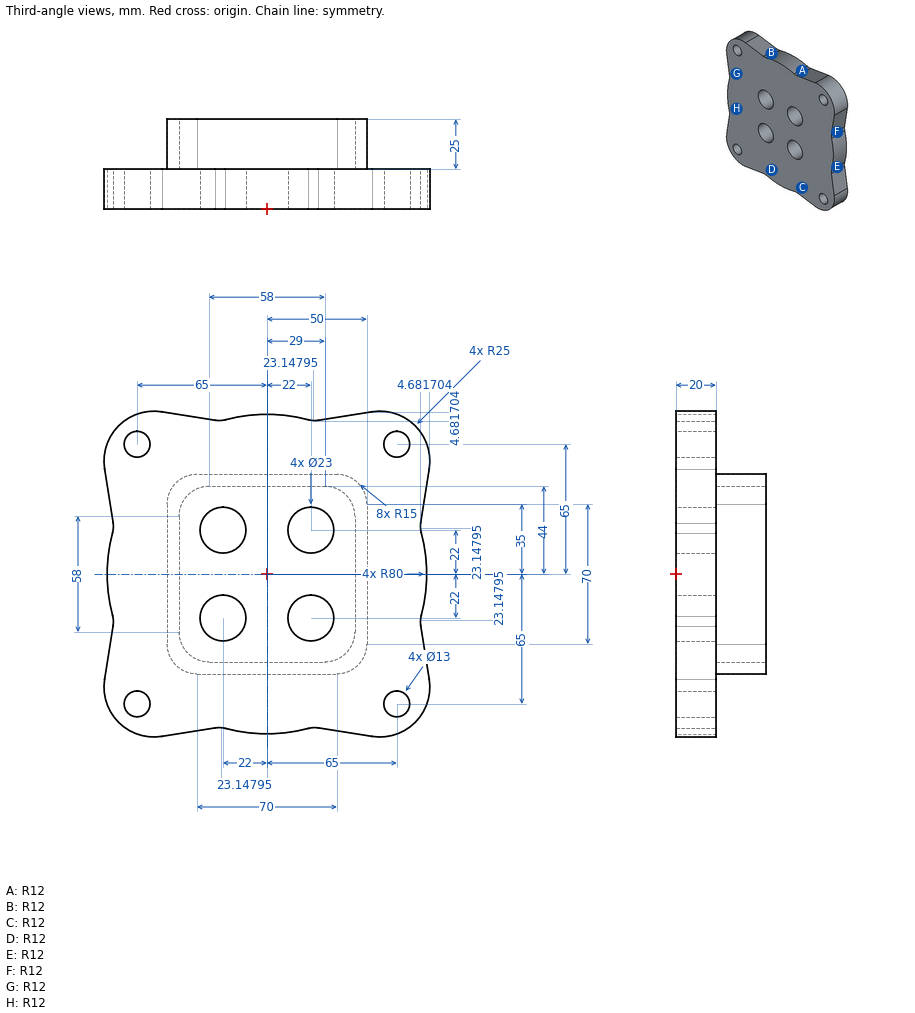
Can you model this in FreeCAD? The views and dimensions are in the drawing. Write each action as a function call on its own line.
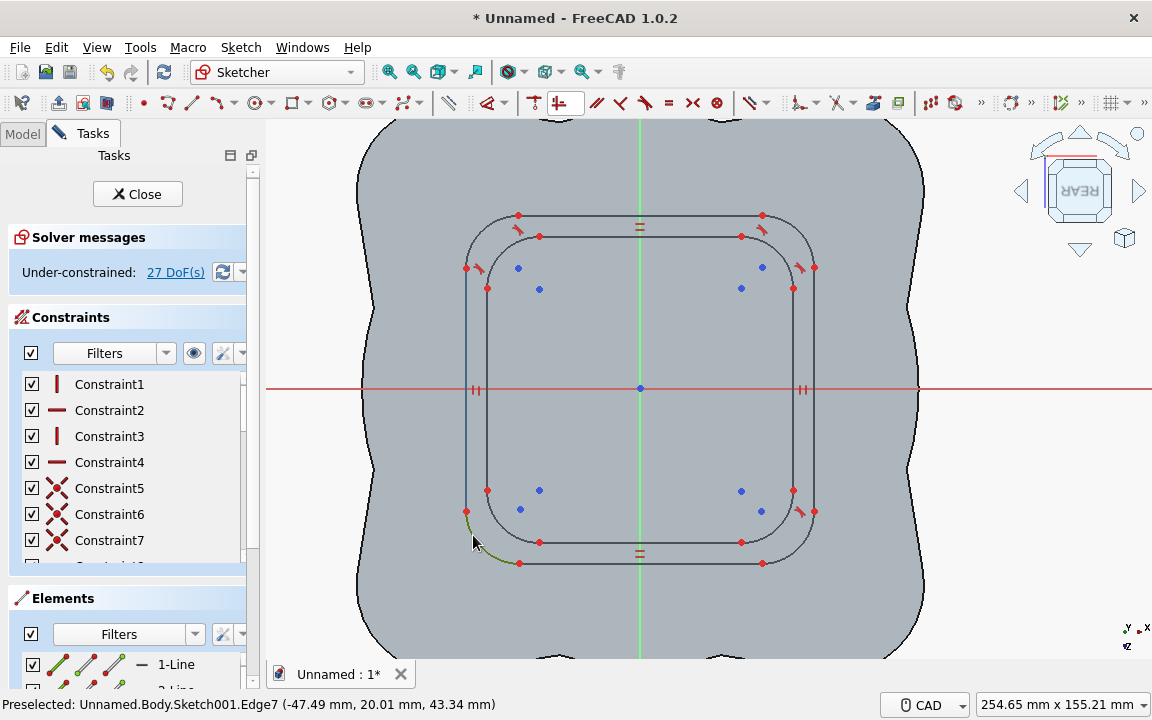
click(646, 104)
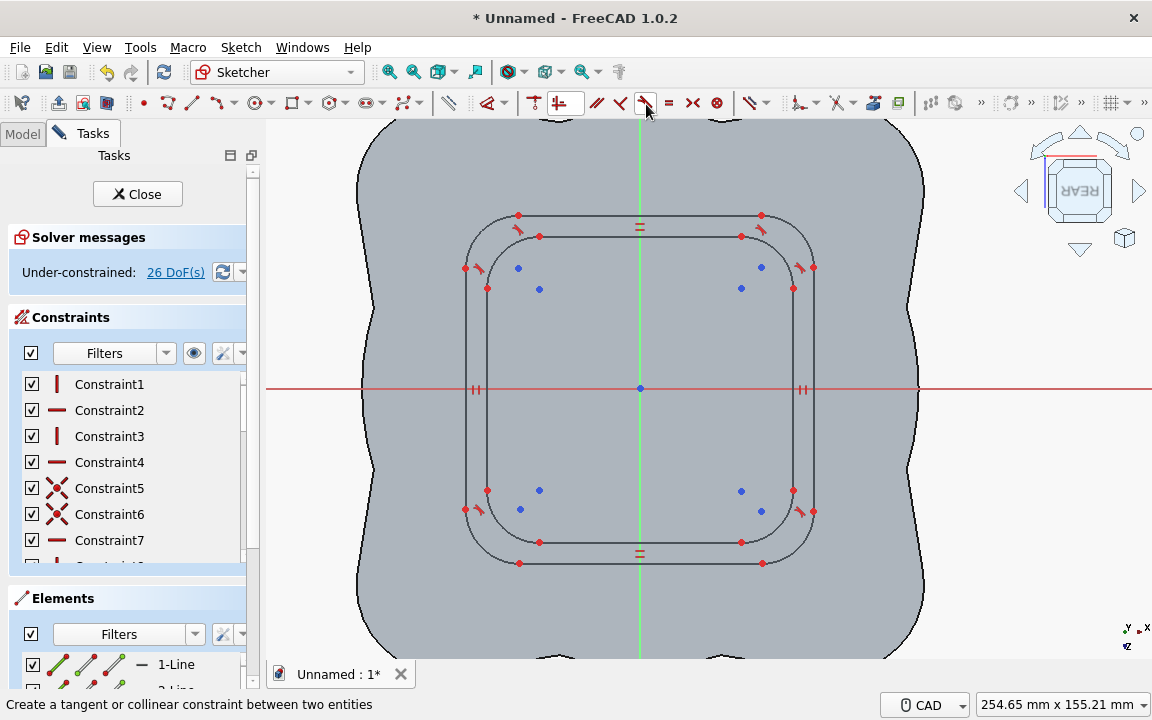
click(592, 564)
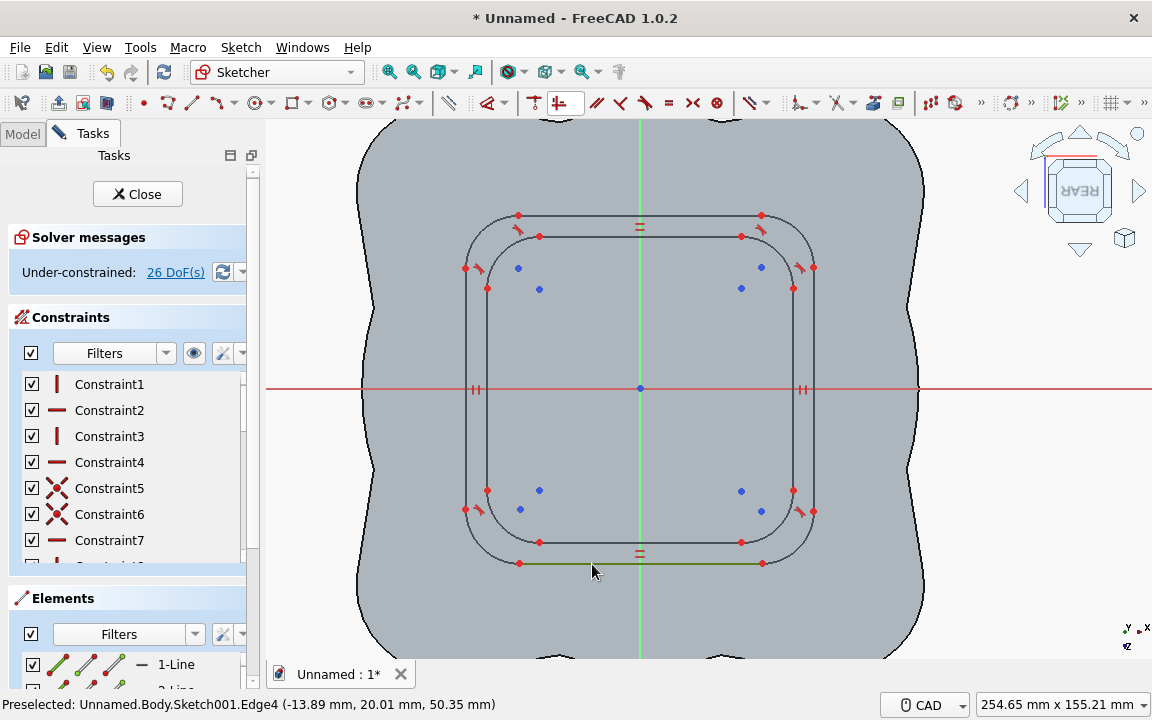
click(472, 534)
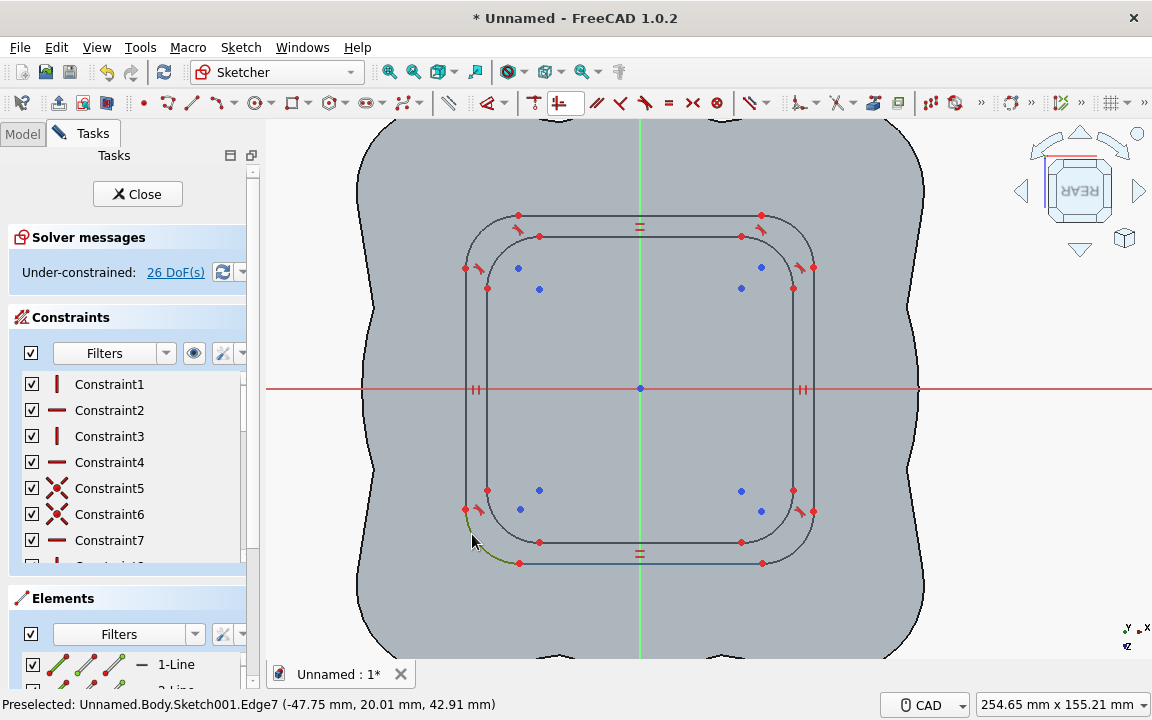
click(646, 104)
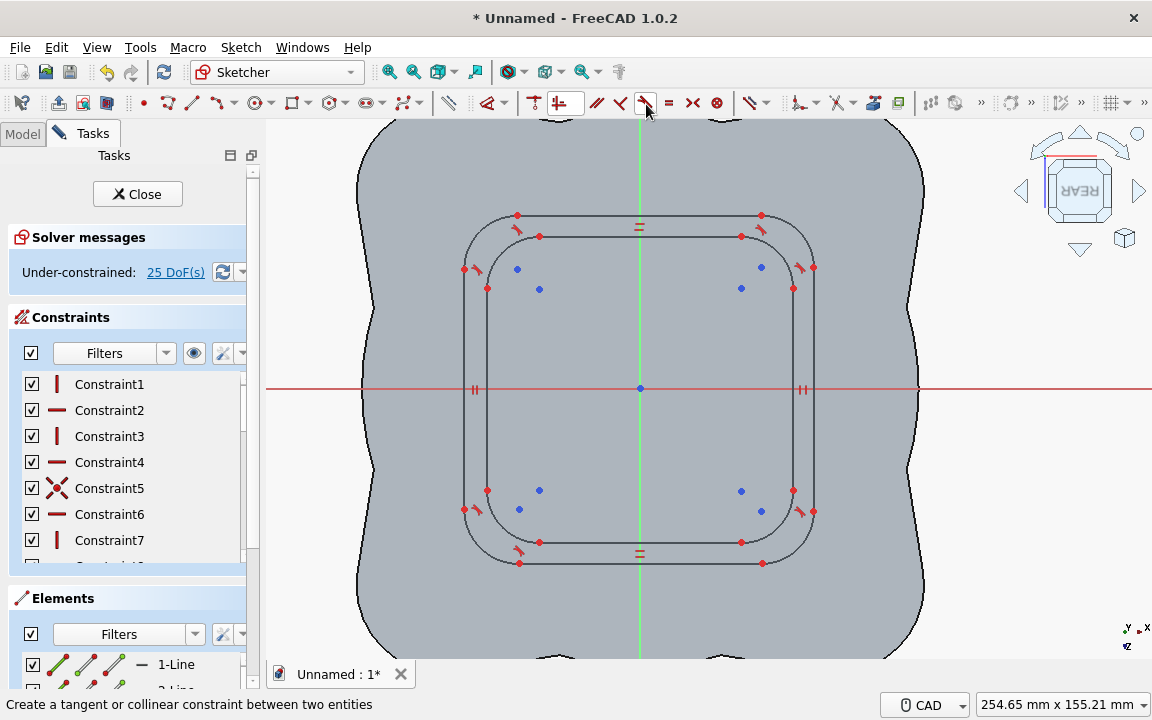
click(592, 564)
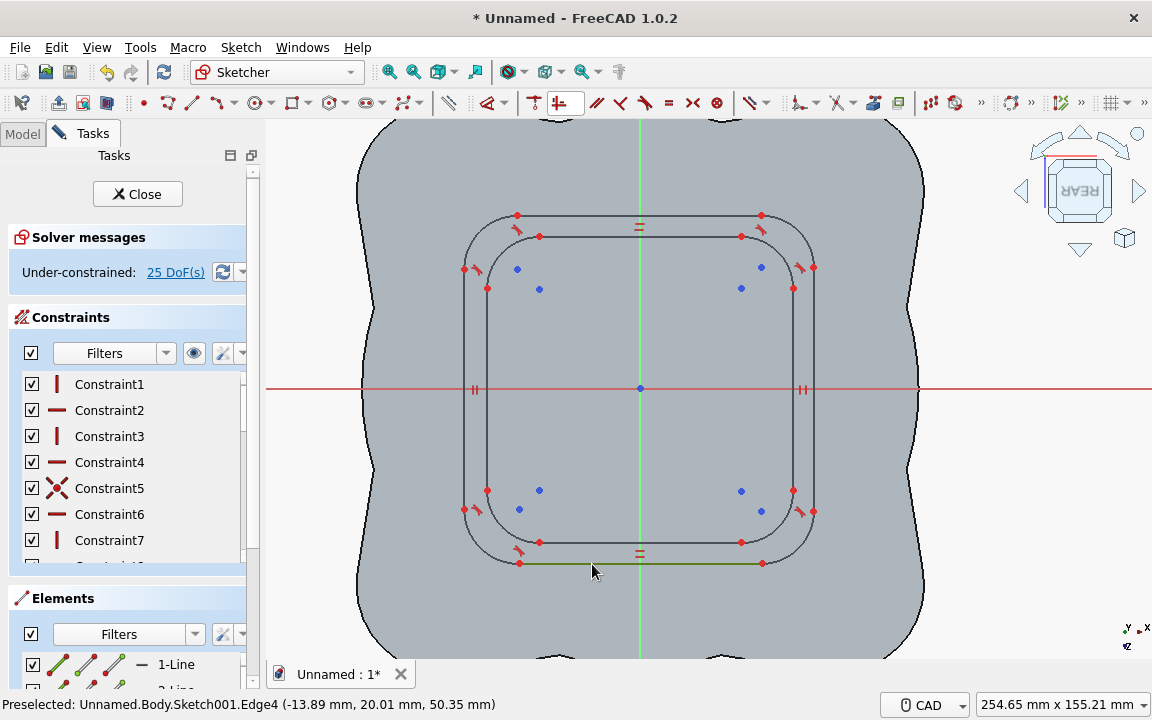
click(786, 558)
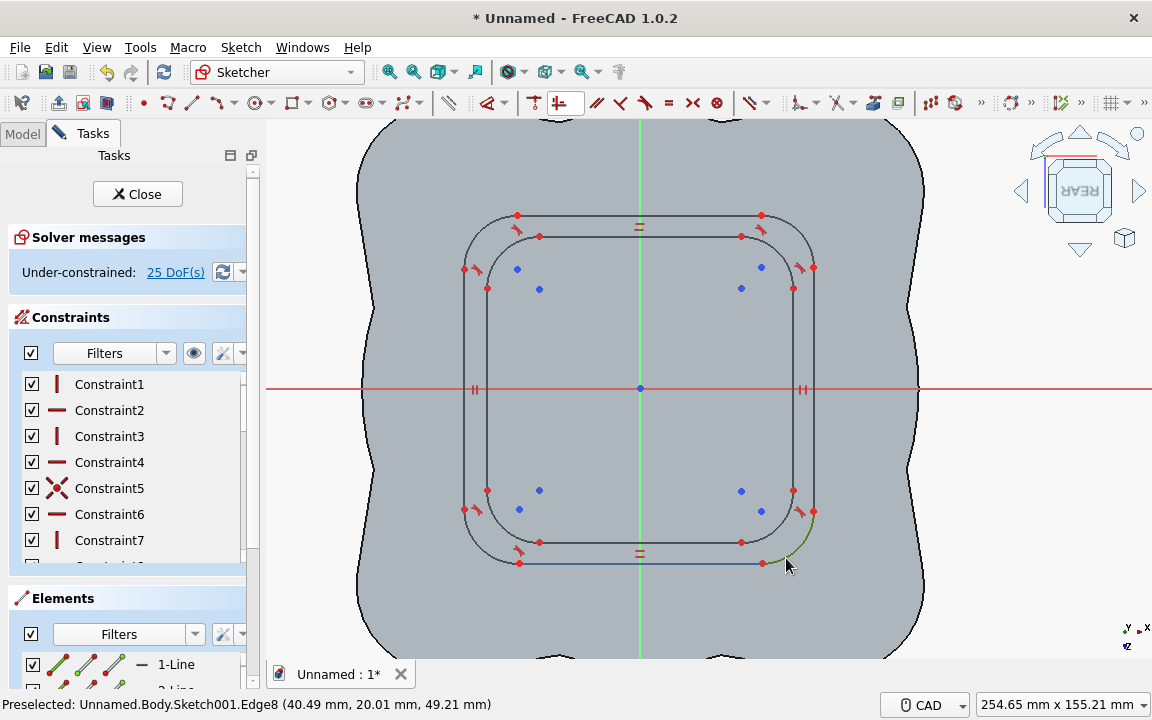
click(646, 104)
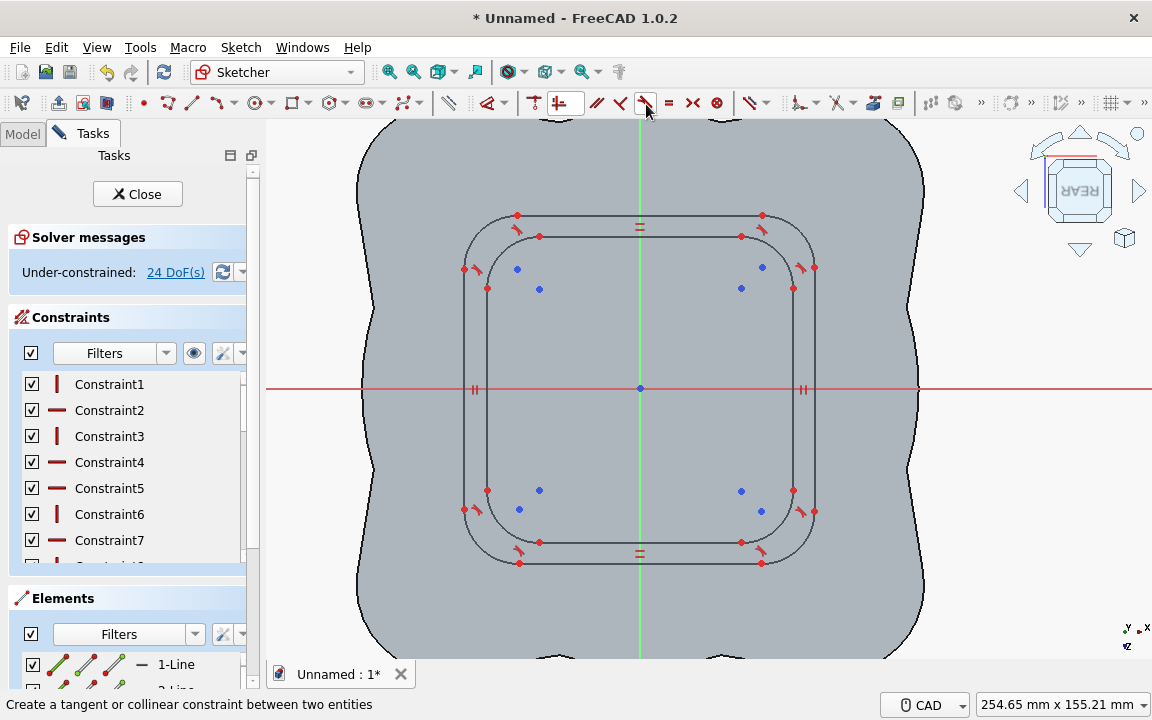
click(680, 543)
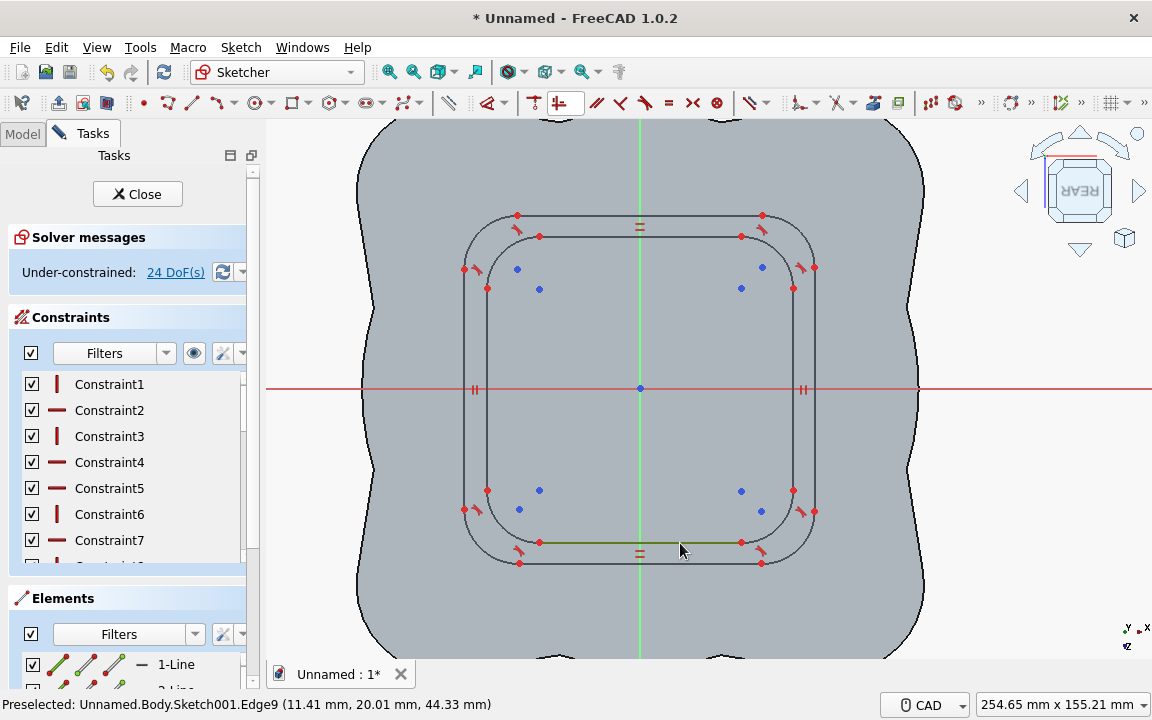
click(493, 514)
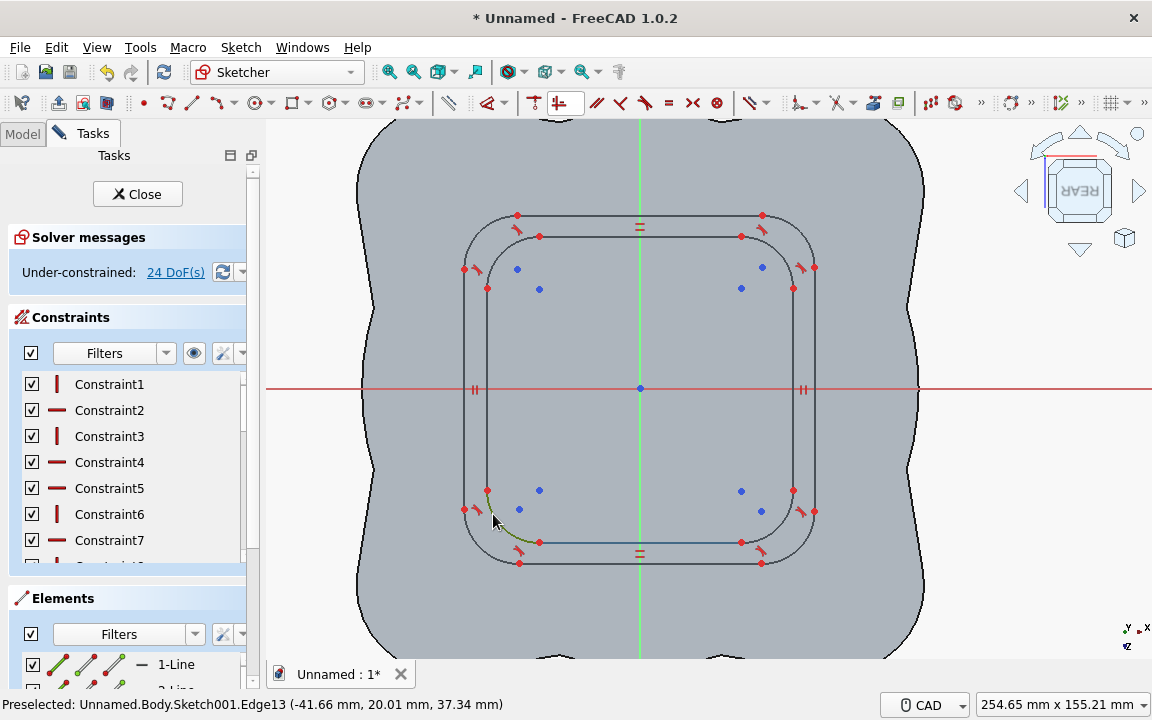
click(646, 104)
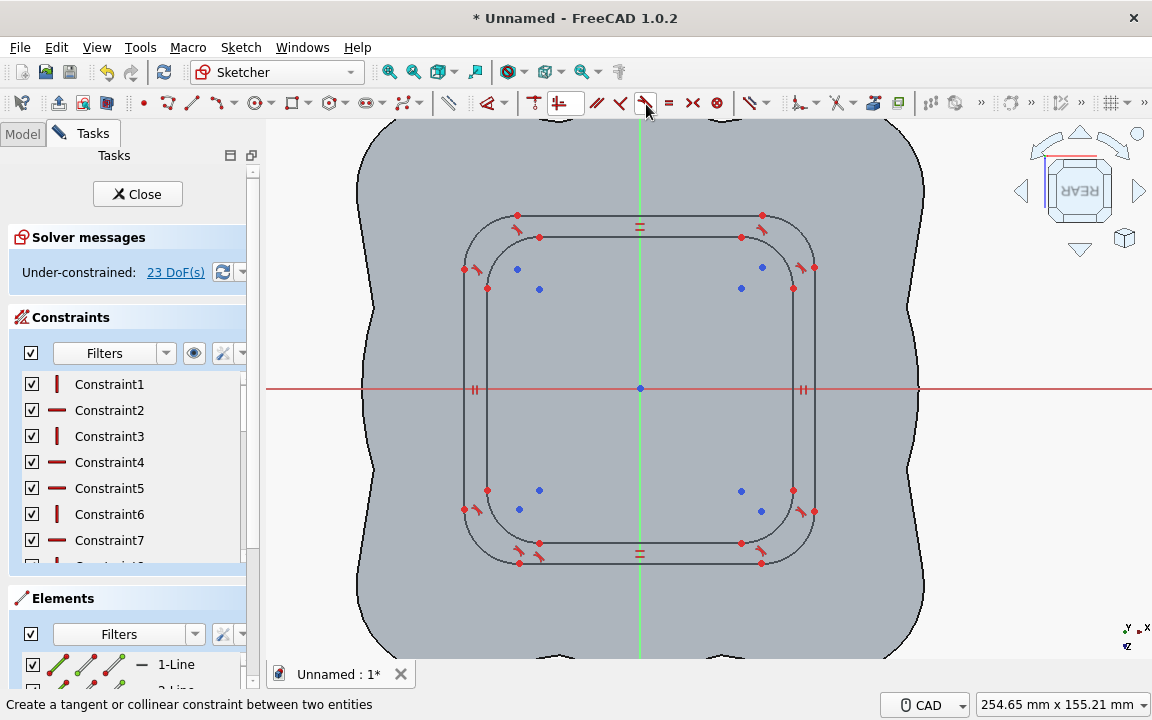
click(681, 543)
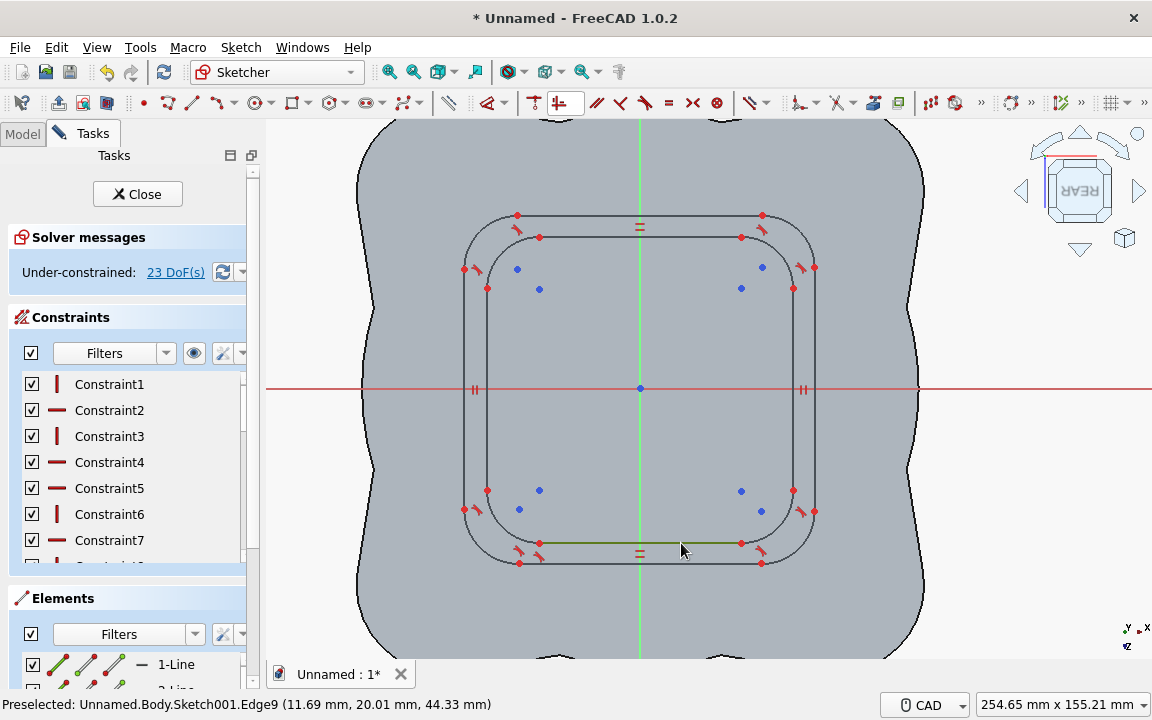
click(765, 538)